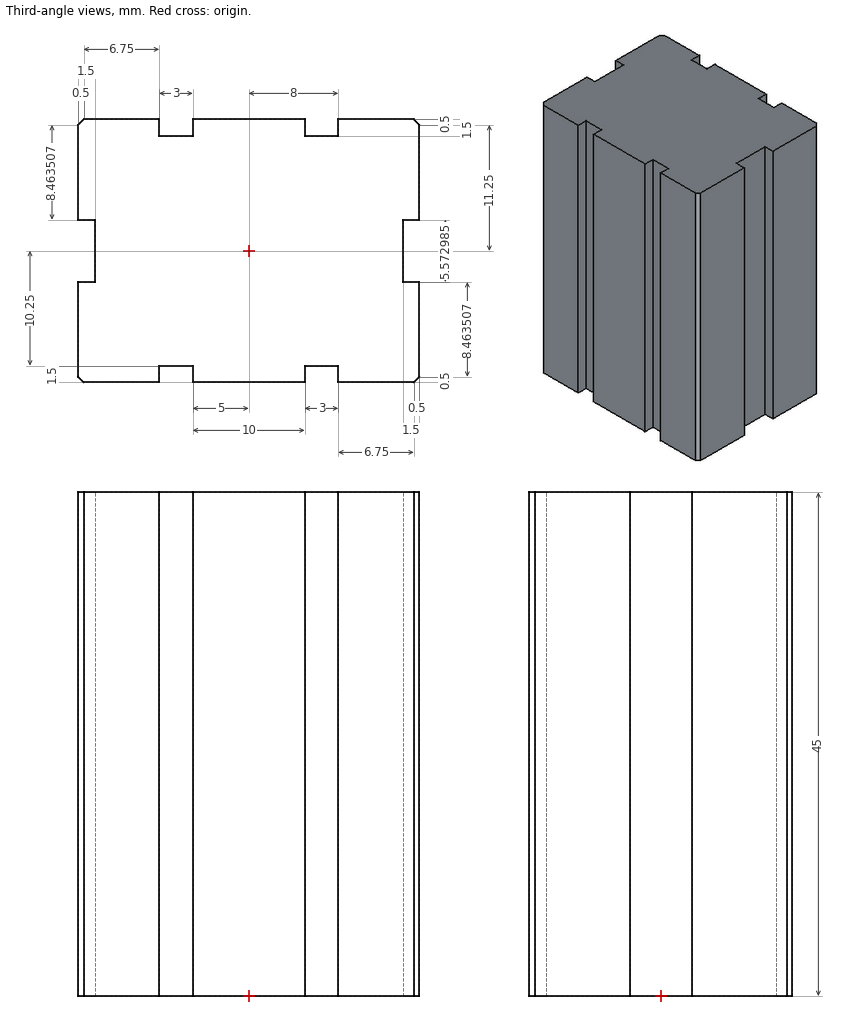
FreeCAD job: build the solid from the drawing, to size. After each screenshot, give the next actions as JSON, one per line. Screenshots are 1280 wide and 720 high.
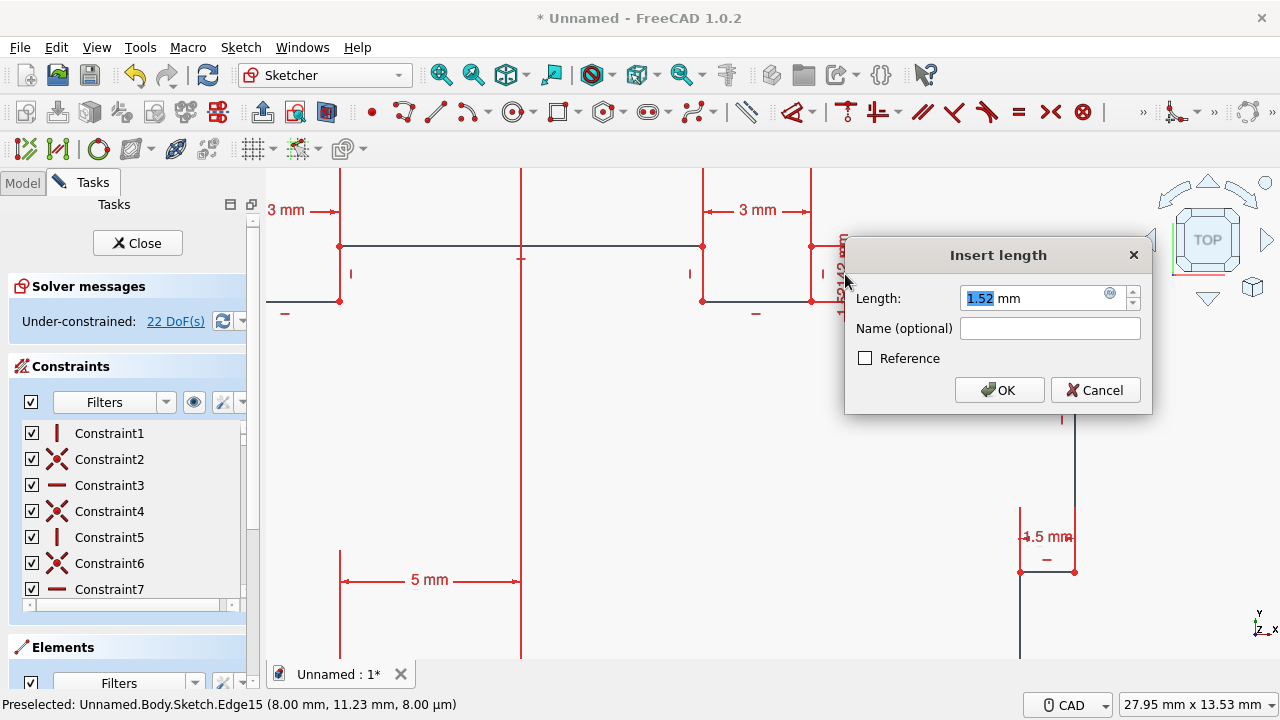
{"action": "type", "text": "1.5"}
{"action": "key", "text": "Return"}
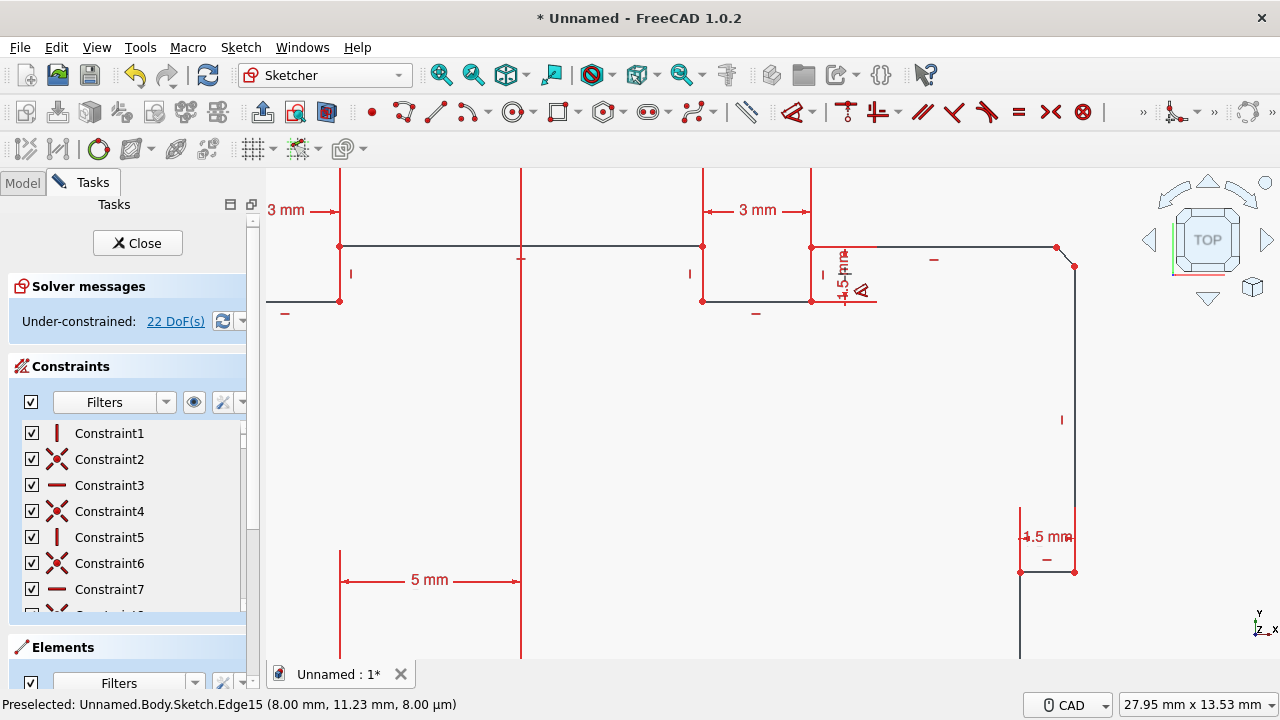
{"action": "left_click", "coordinate": [703, 285]}
{"action": "left_click", "coordinate": [737, 274]}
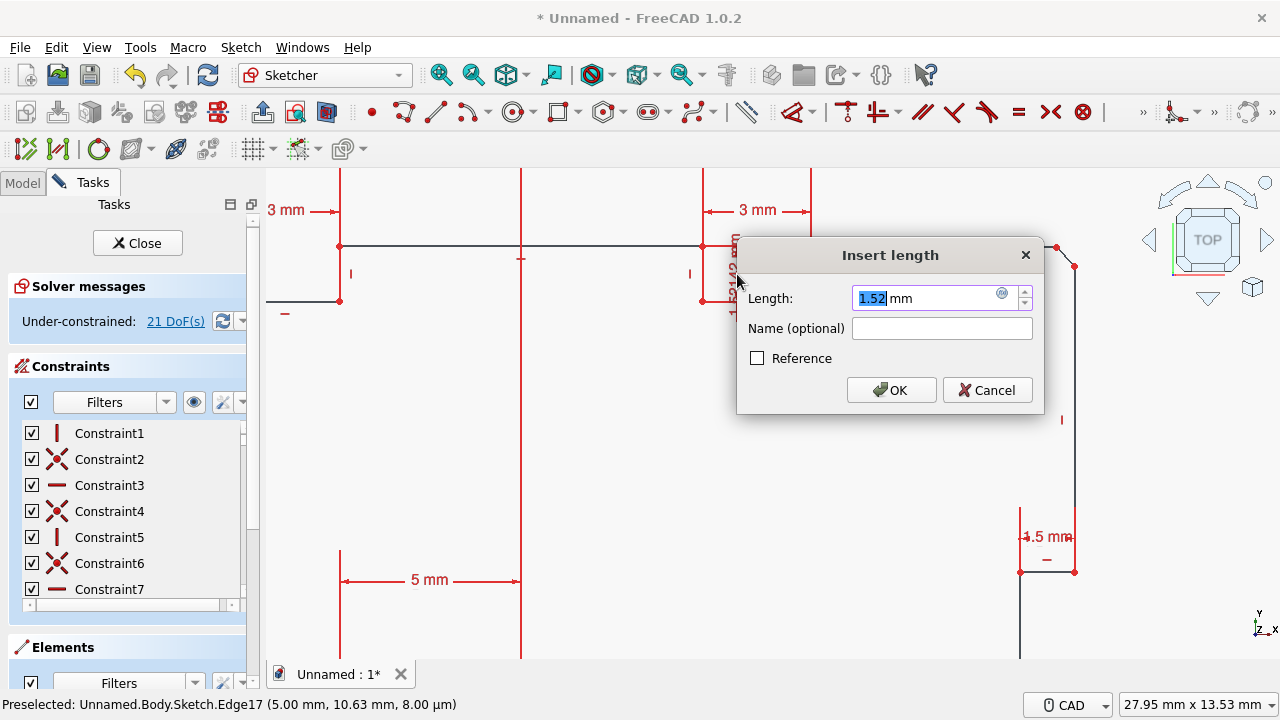
{"action": "type", "text": "1.5"}
{"action": "key", "text": "Return"}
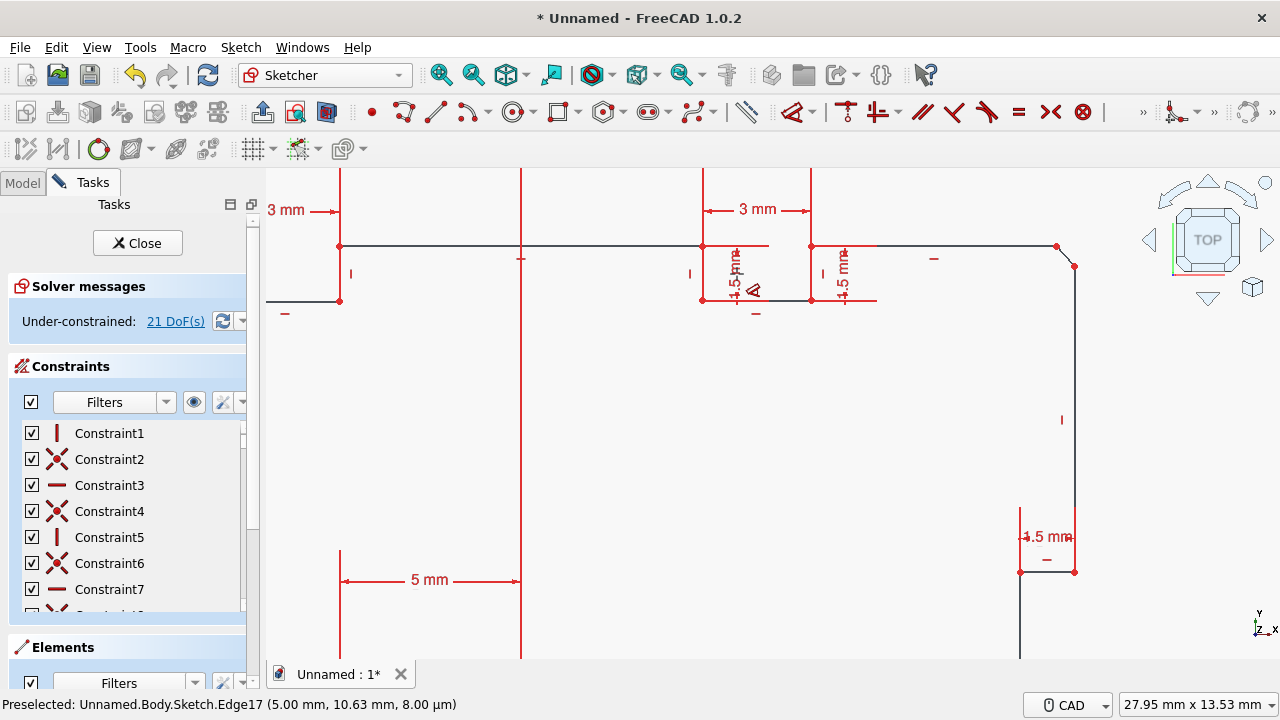
{"action": "left_click", "coordinate": [340, 263]}
{"action": "left_click", "coordinate": [306, 274]}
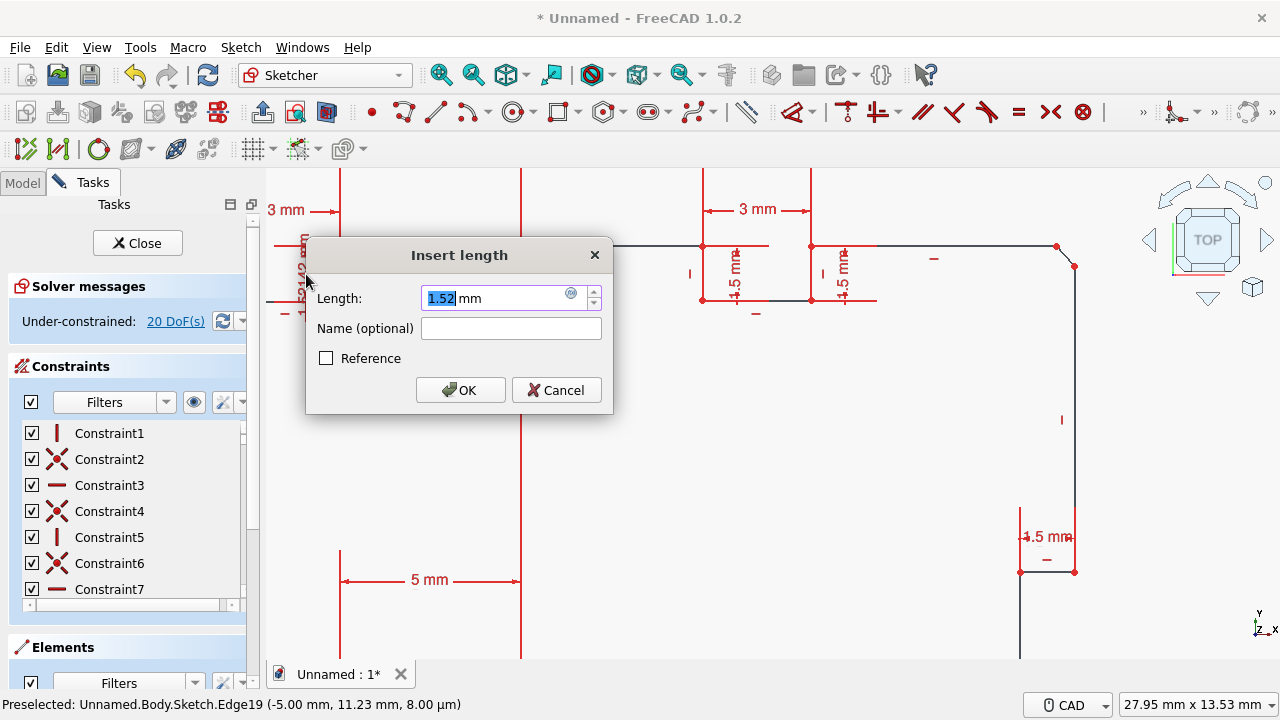
{"action": "type", "text": "1.5"}
{"action": "key", "text": "Return"}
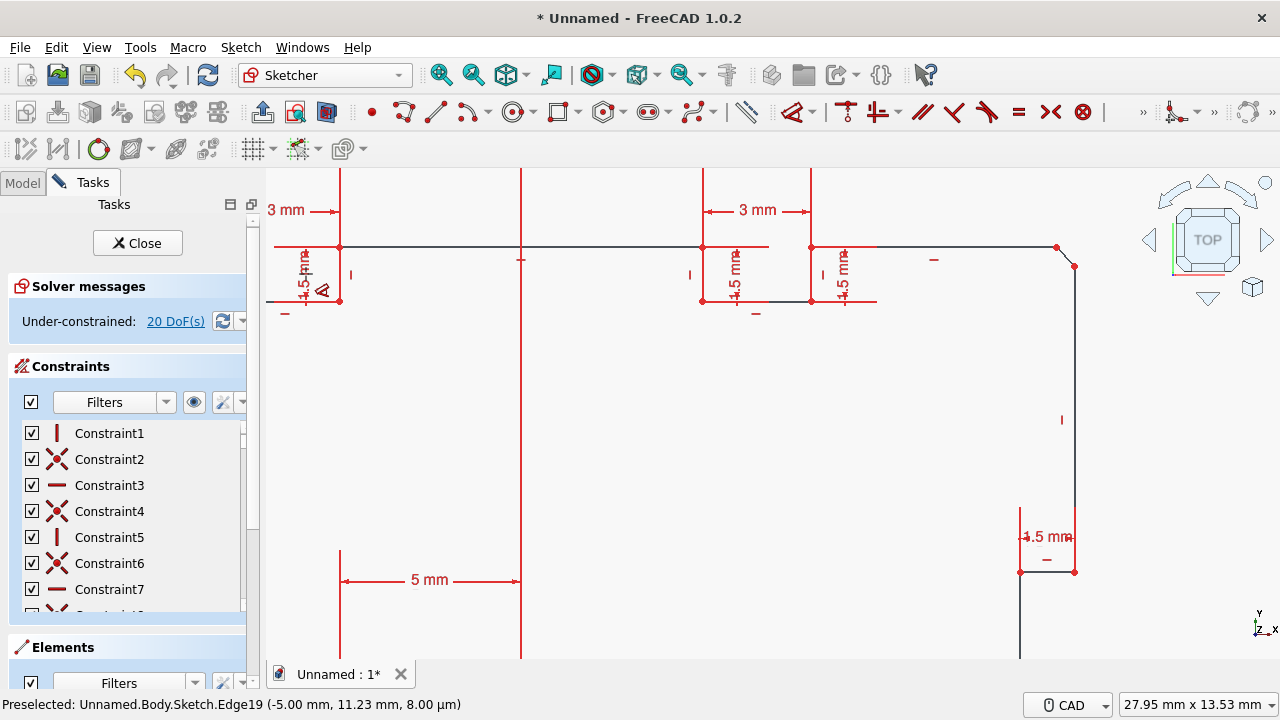
{"action": "scroll", "coordinate": [811, 263], "scroll_direction": "down", "scroll_amount": 5}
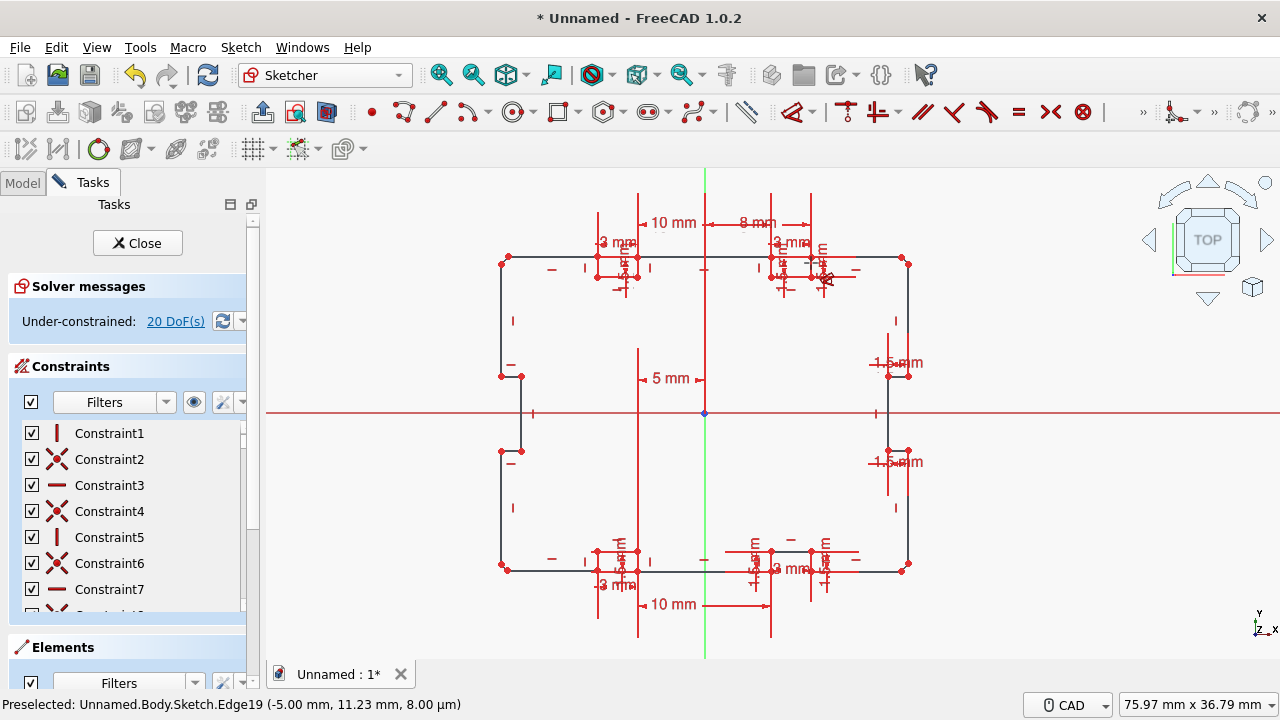
{"action": "scroll", "coordinate": [598, 271], "scroll_direction": "up", "scroll_amount": 5}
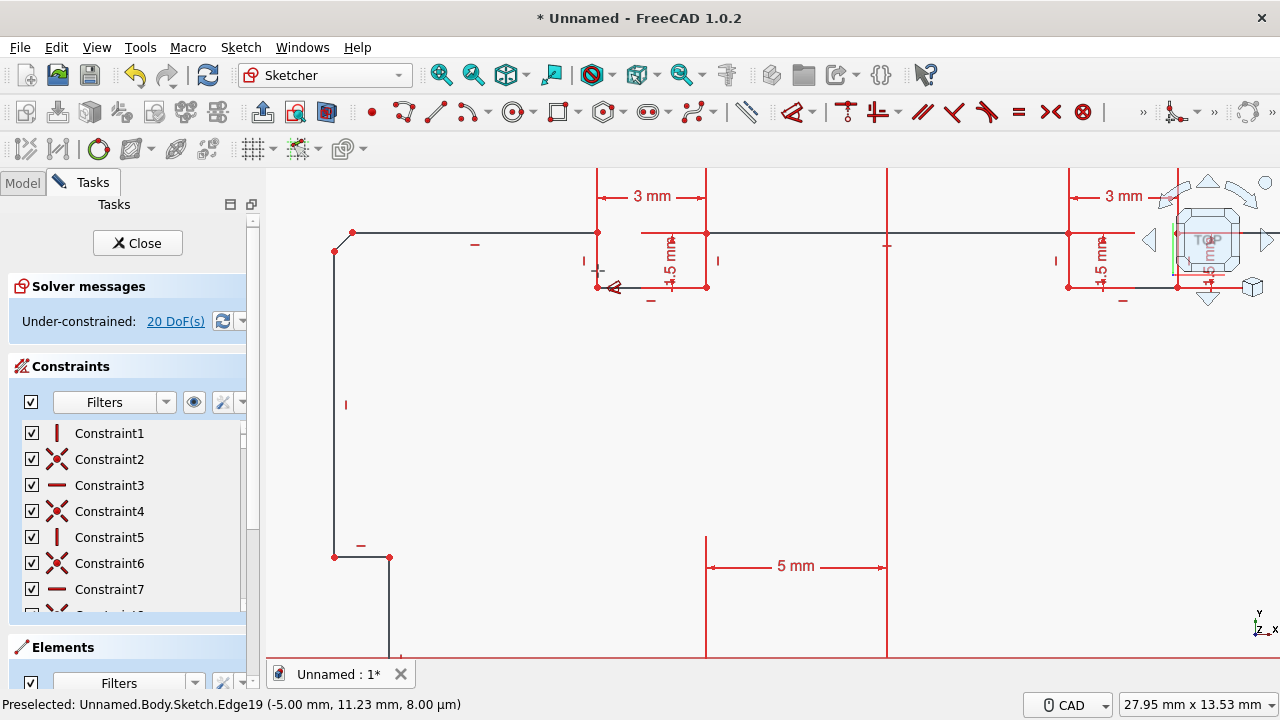
{"action": "left_click", "coordinate": [597, 271]}
{"action": "left_click", "coordinate": [563, 260]}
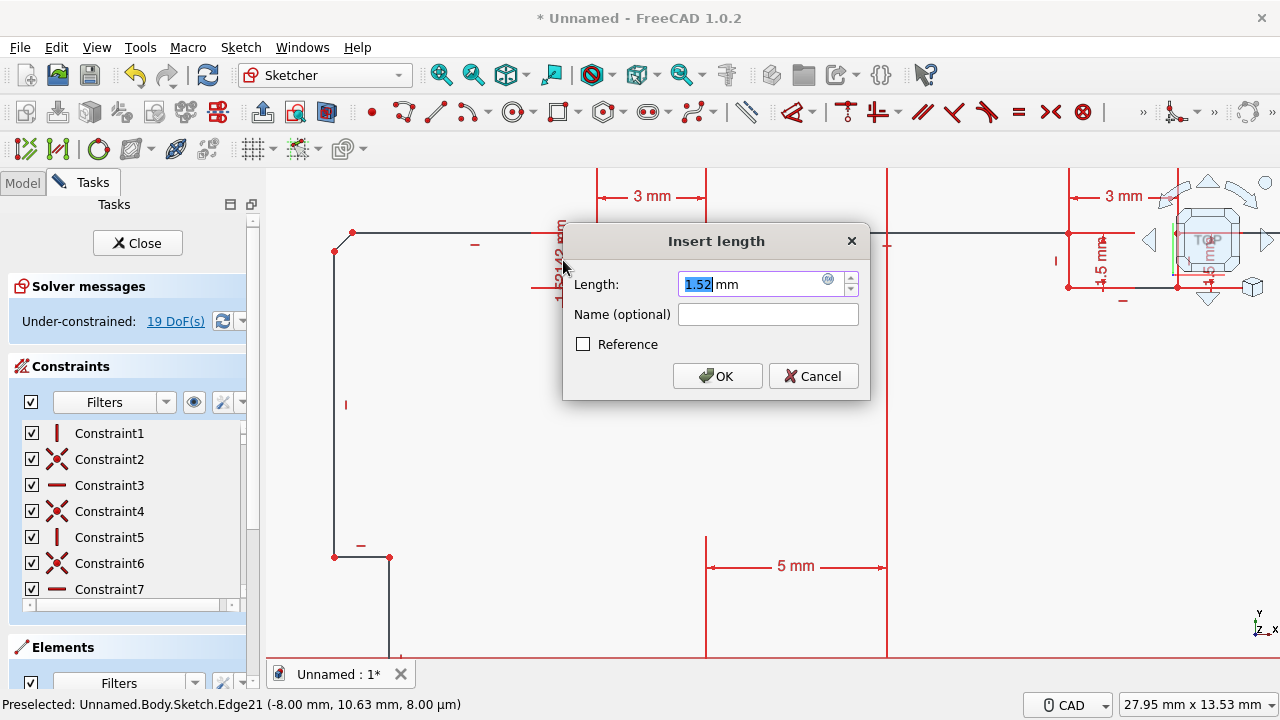
{"action": "type", "text": "1.5"}
{"action": "key", "text": "Return"}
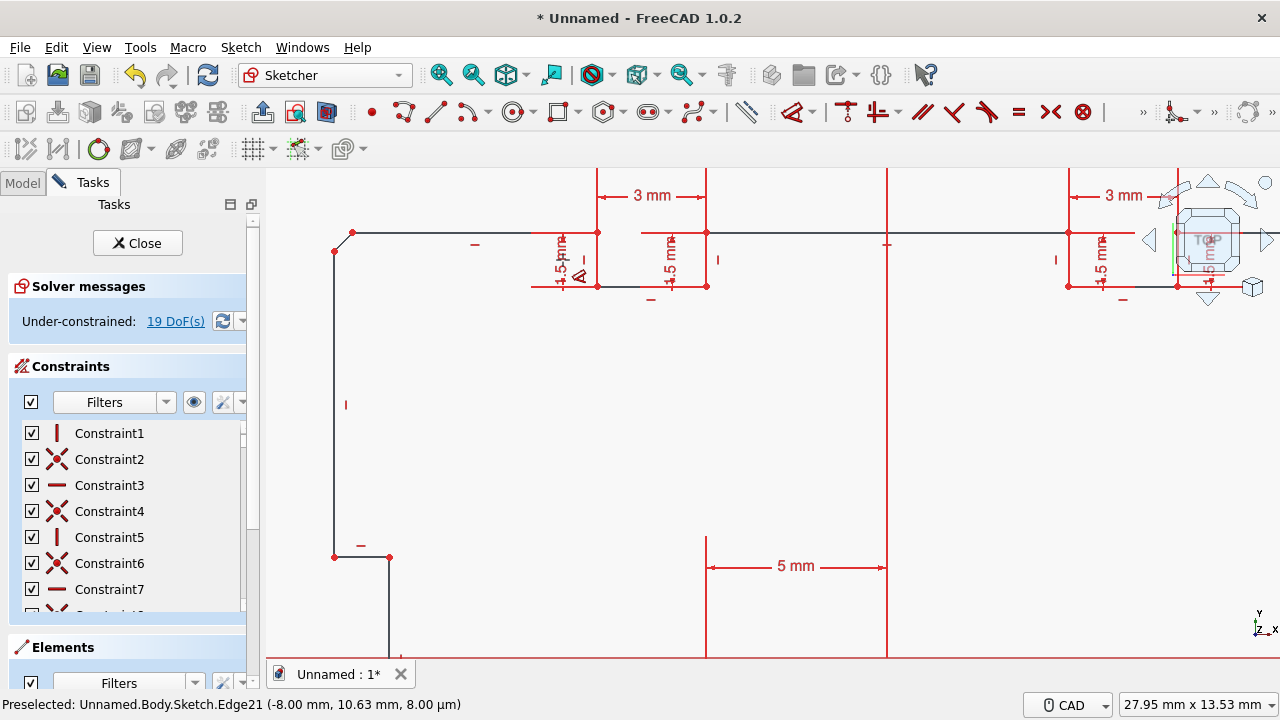
{"action": "left_click", "coordinate": [351, 557]}
{"action": "left_click", "coordinate": [362, 523]}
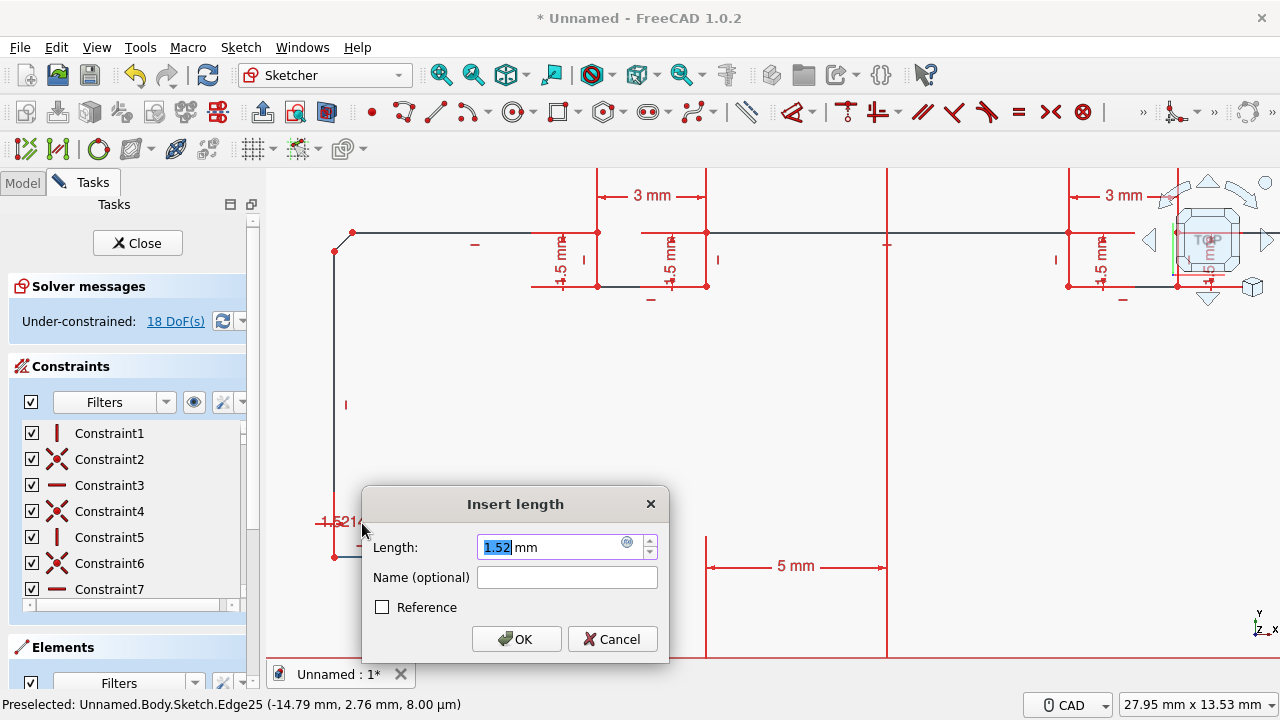
{"action": "type", "text": "1.5"}
{"action": "key", "text": "Return"}